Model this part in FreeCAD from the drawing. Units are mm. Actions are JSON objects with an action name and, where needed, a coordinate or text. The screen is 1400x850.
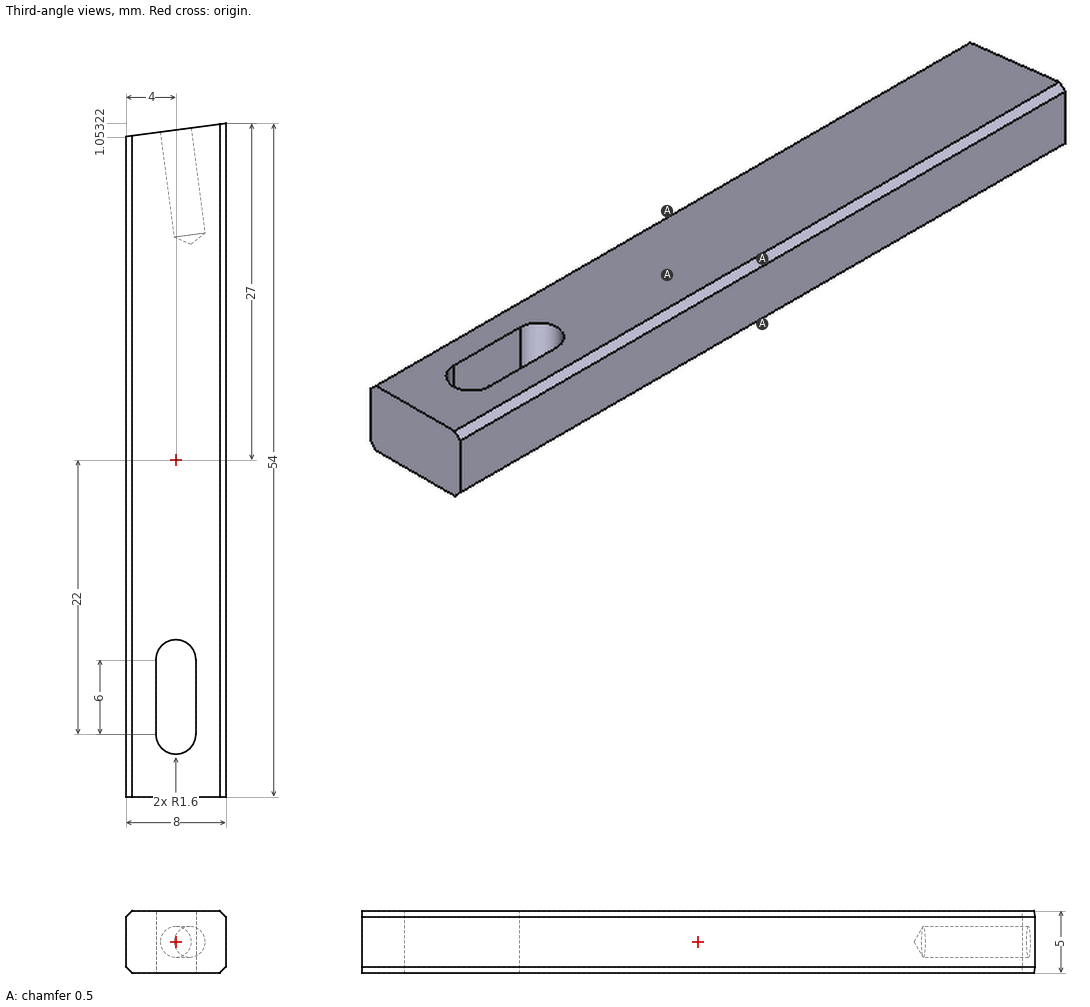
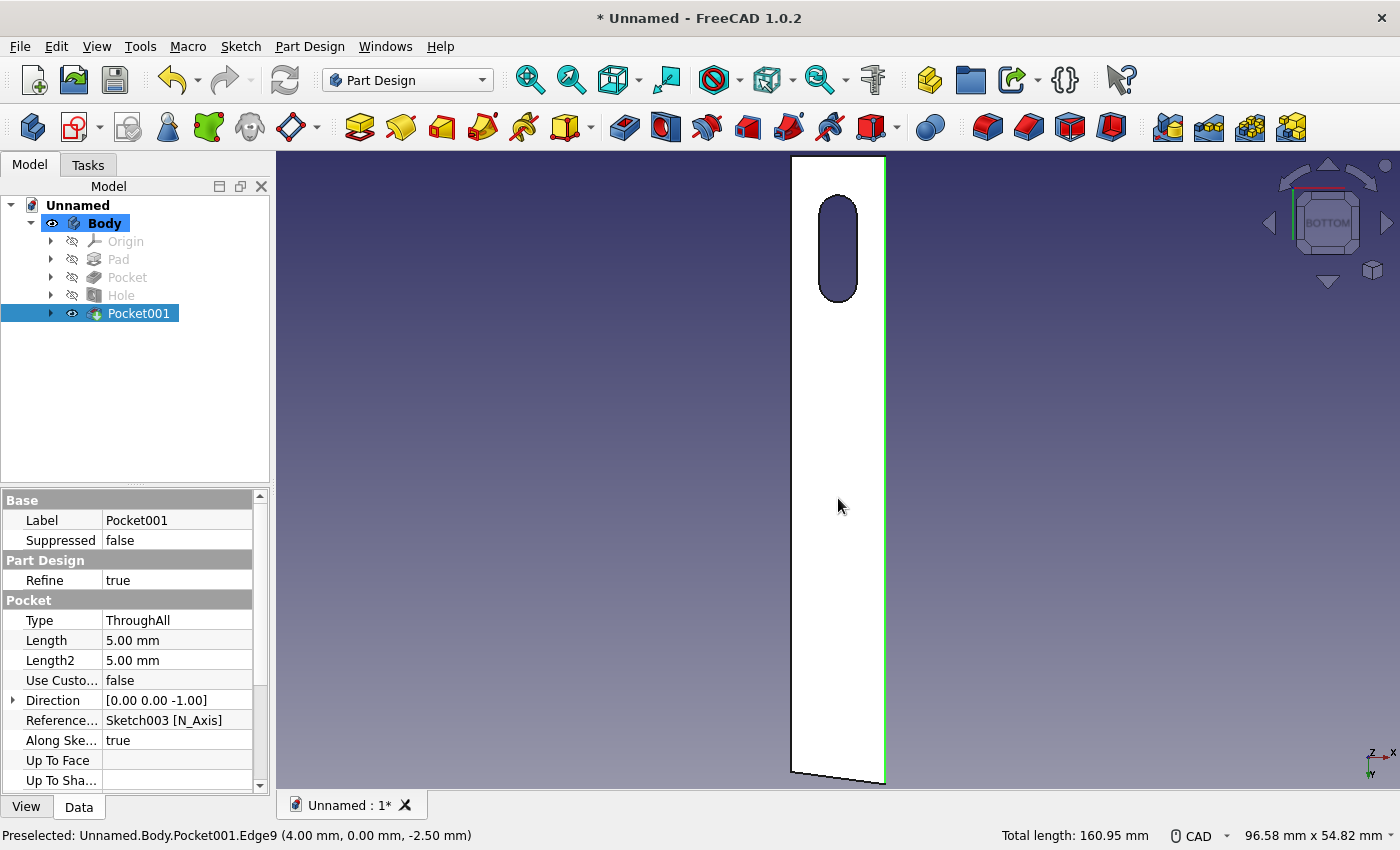
{"action": "left_click", "coordinate": [791, 463], "text": "ctrl"}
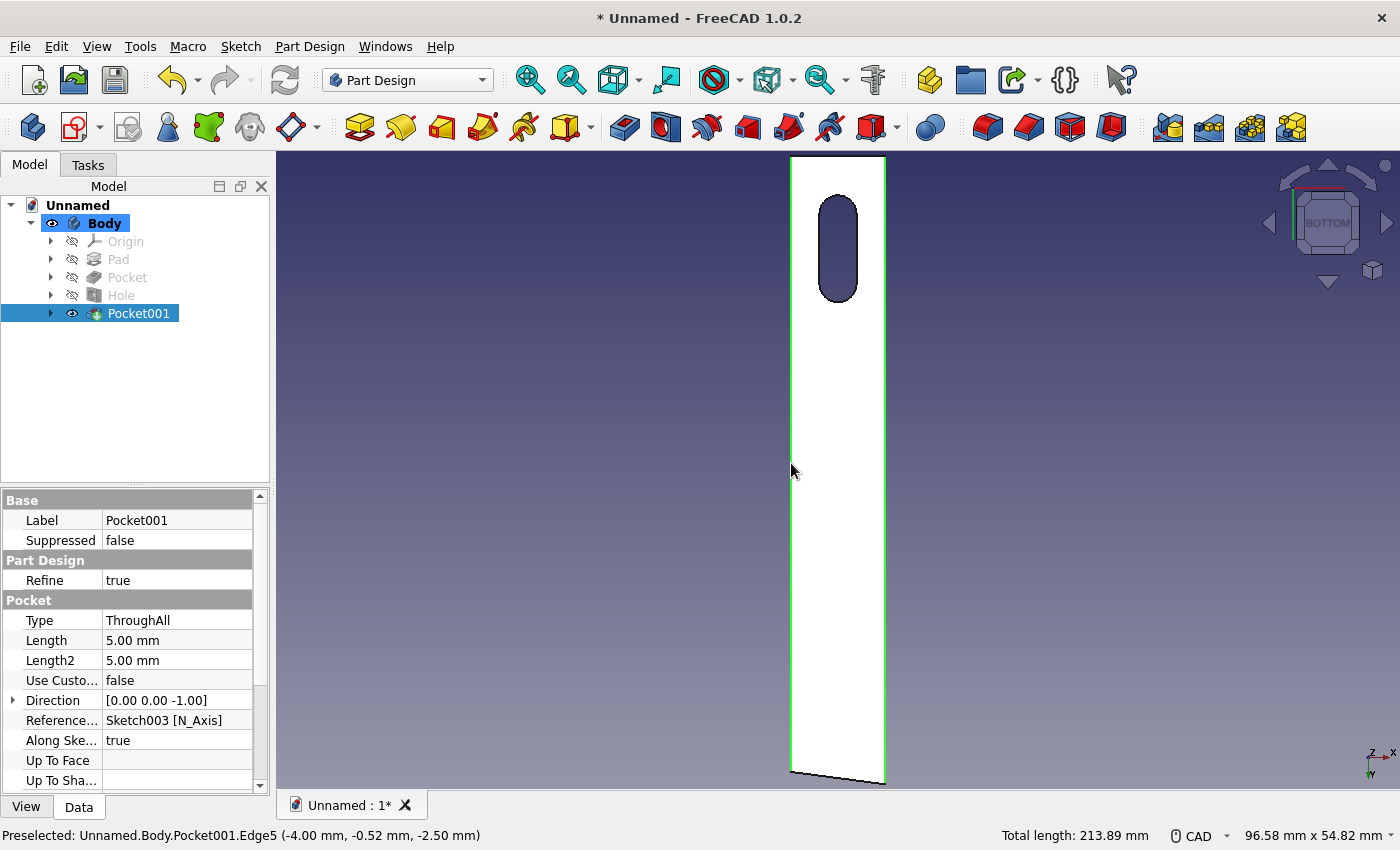
{"action": "left_click", "coordinate": [1029, 128]}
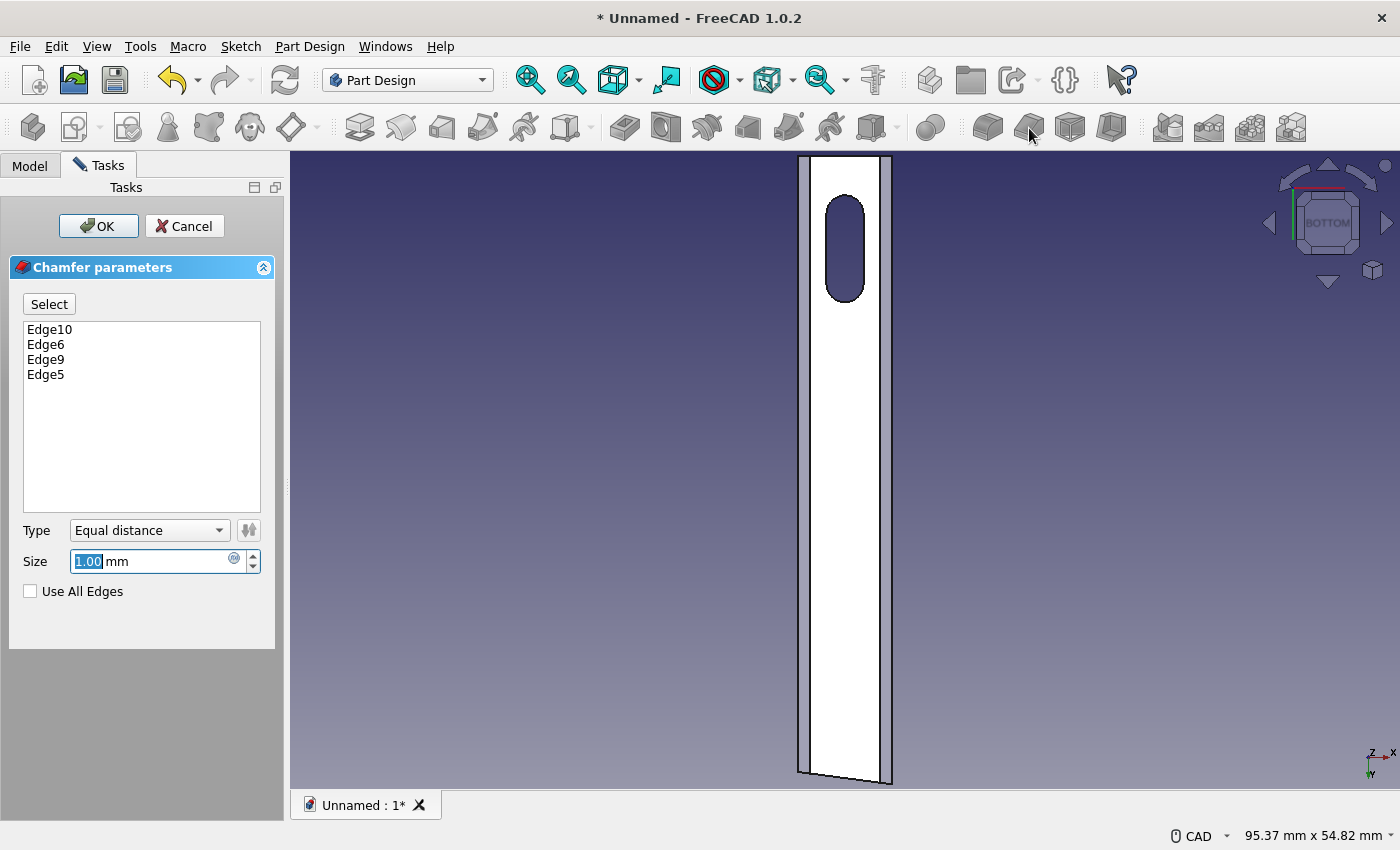
{"action": "type", "text": "0.5"}
{"action": "key", "text": "Tab"}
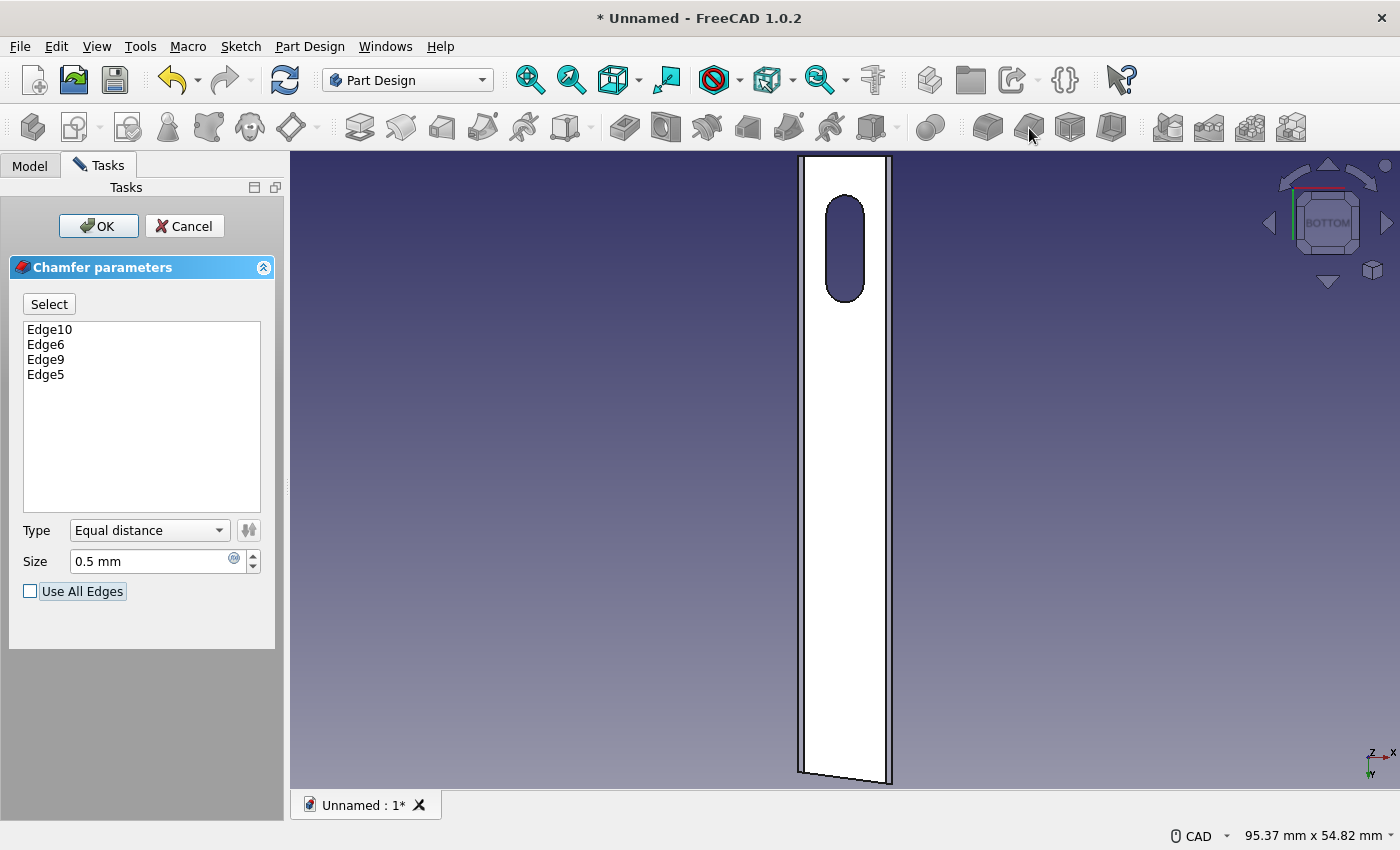
{"action": "left_click", "coordinate": [99, 226]}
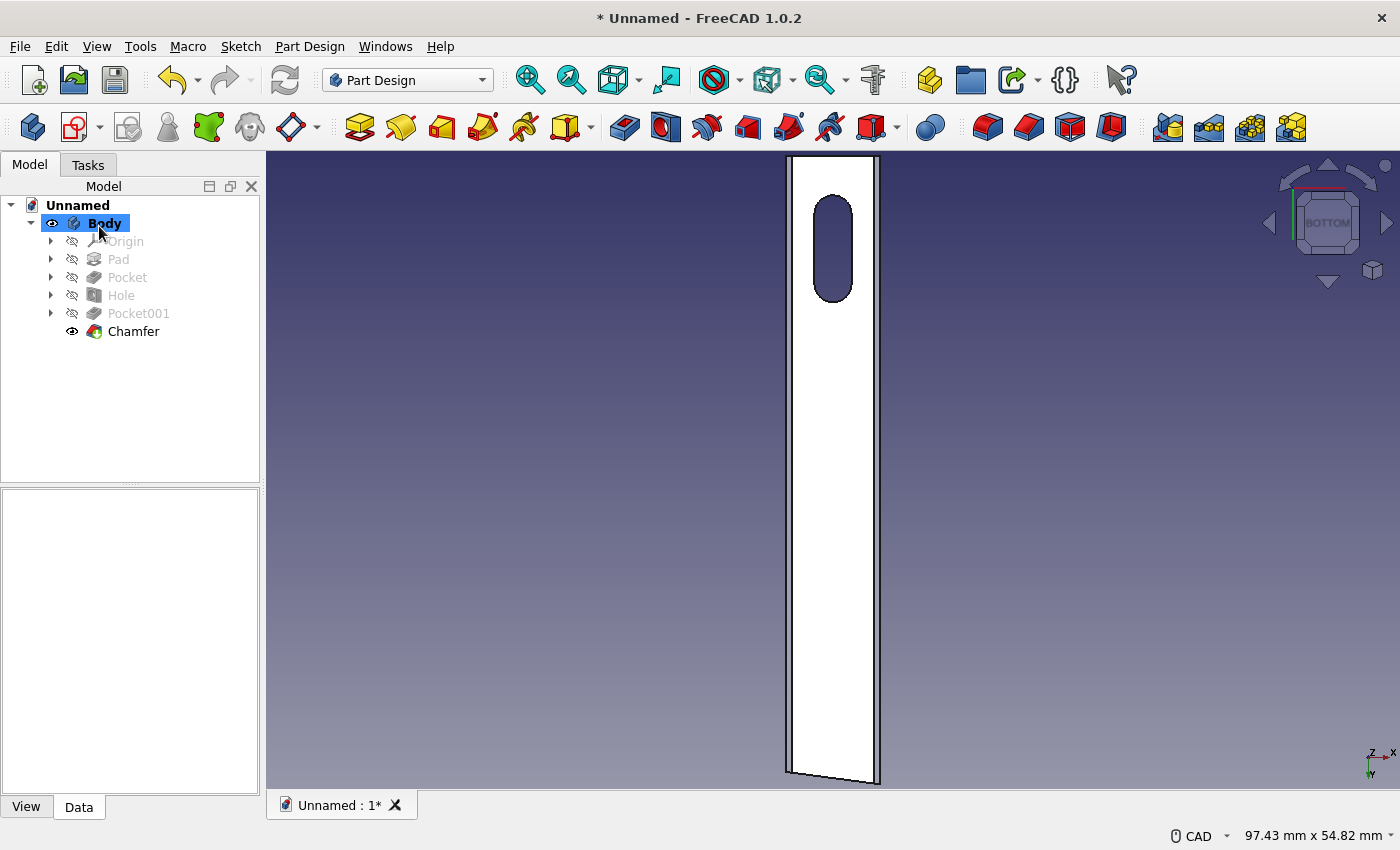
{"action": "key", "text": "0"}